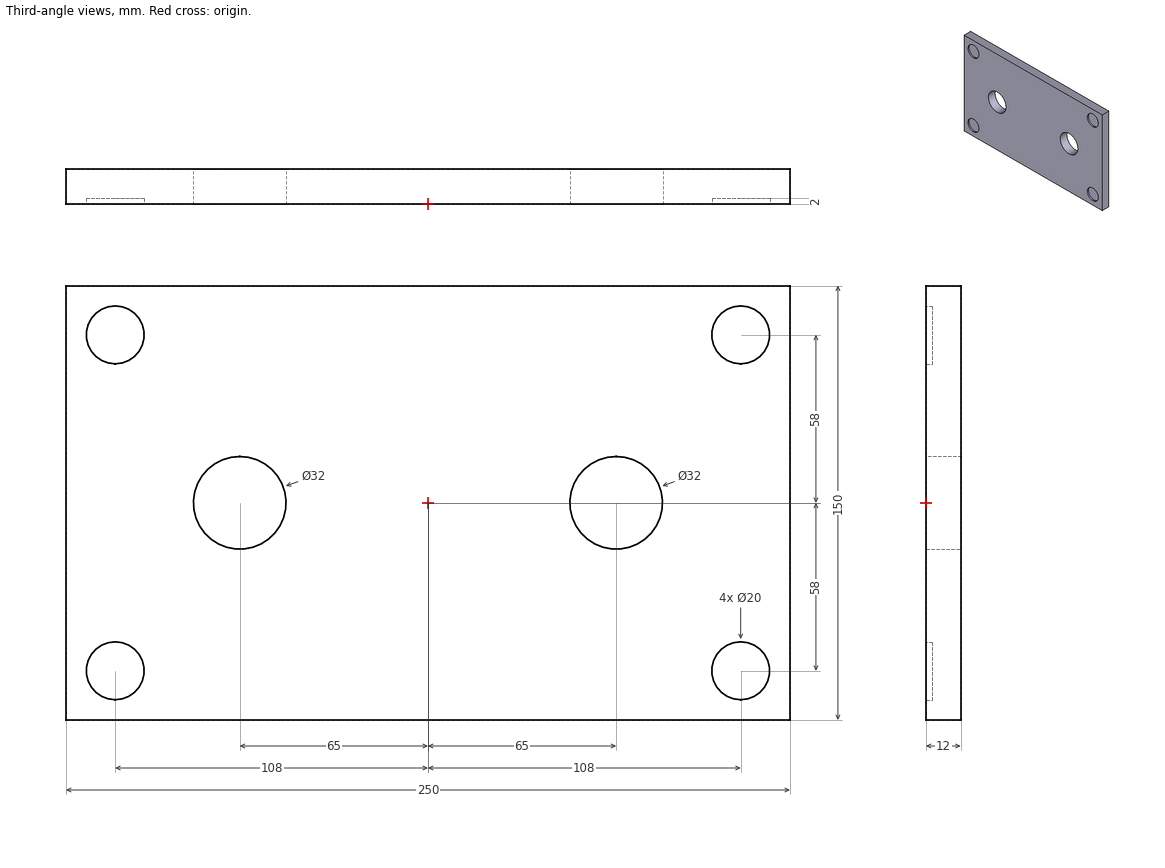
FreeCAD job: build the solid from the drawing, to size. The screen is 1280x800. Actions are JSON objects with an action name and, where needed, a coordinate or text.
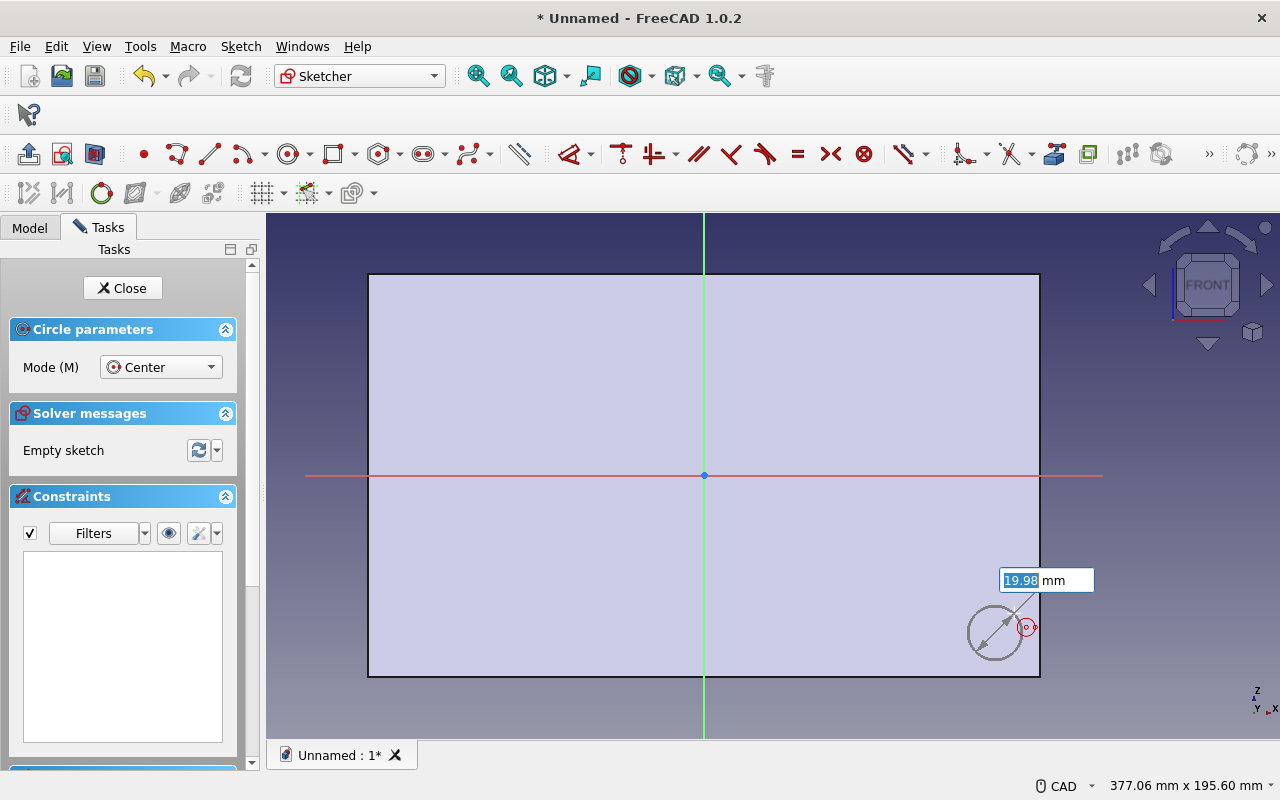
{"action": "type", "text": "20"}
{"action": "key", "text": "Return"}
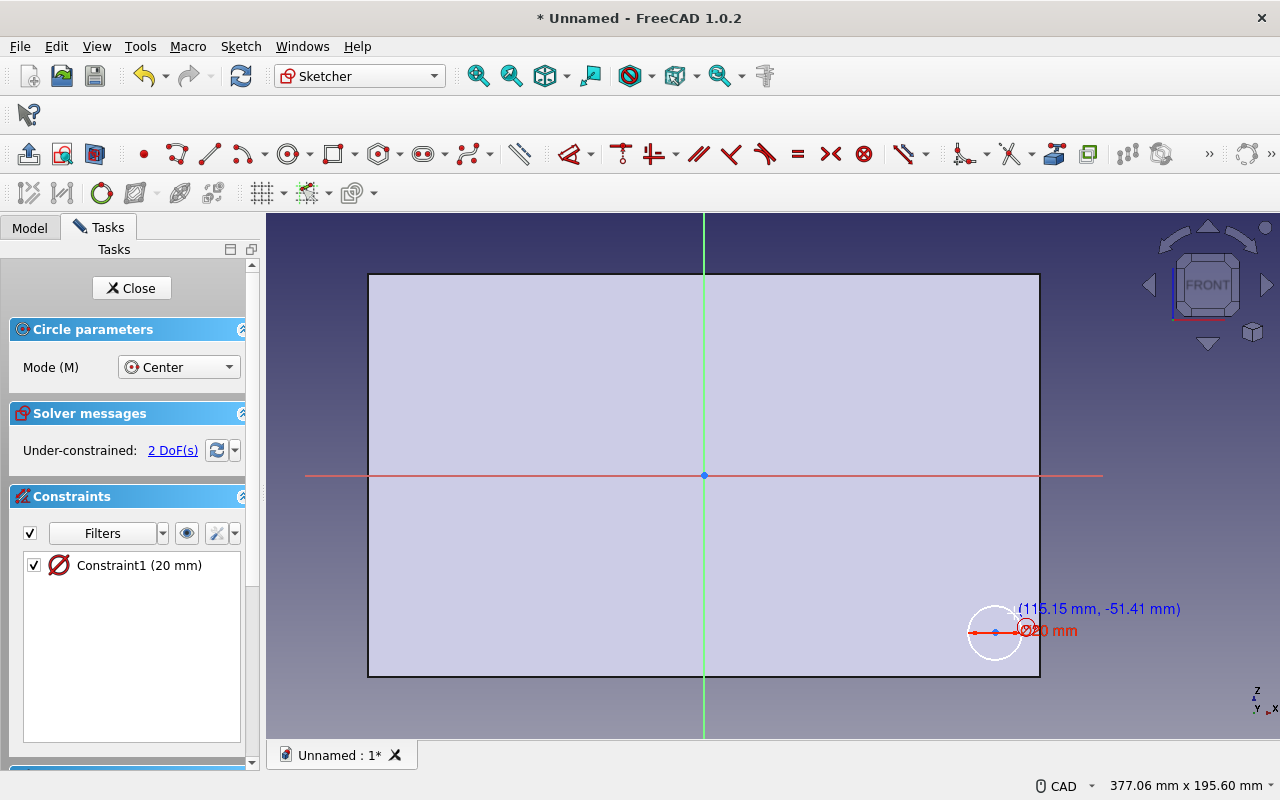
{"action": "left_click", "coordinate": [414, 632]}
{"action": "mouse_move", "coordinate": [433, 613]}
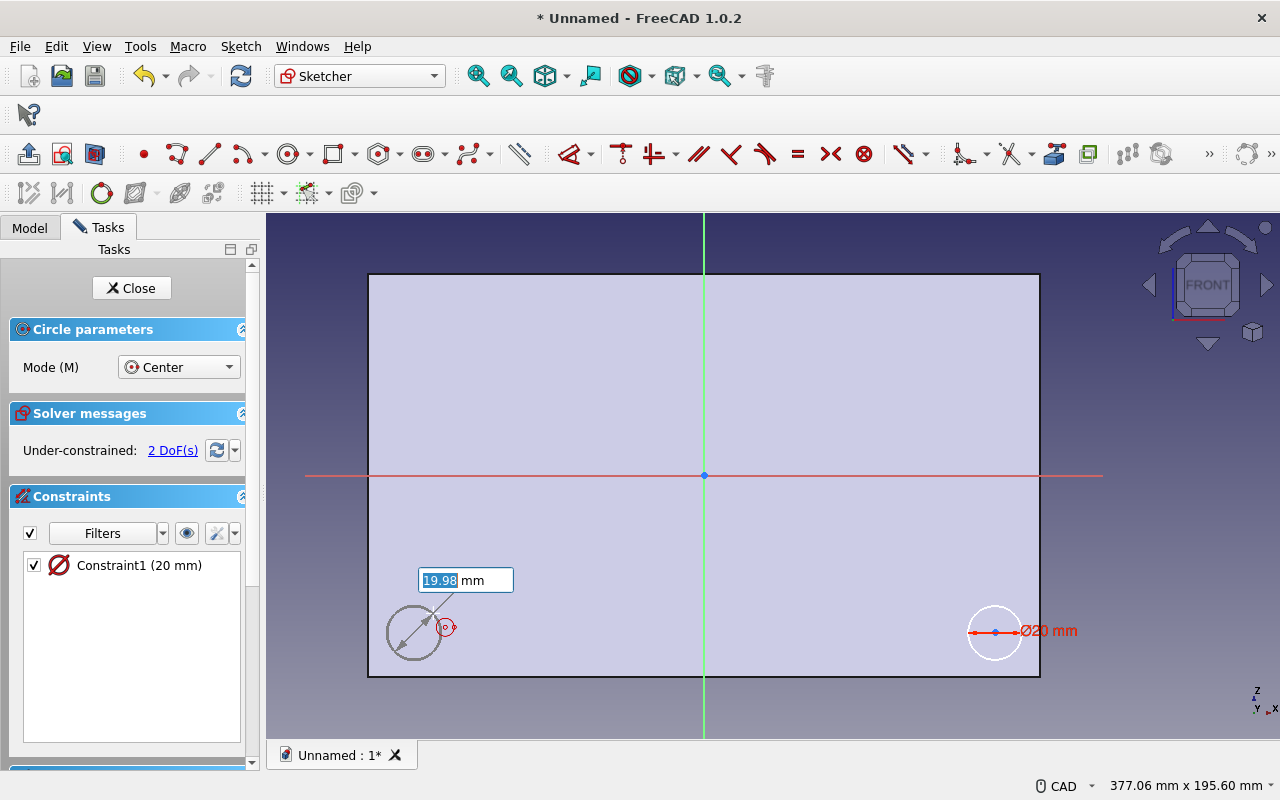
{"action": "type", "text": "20"}
{"action": "key", "text": "Return"}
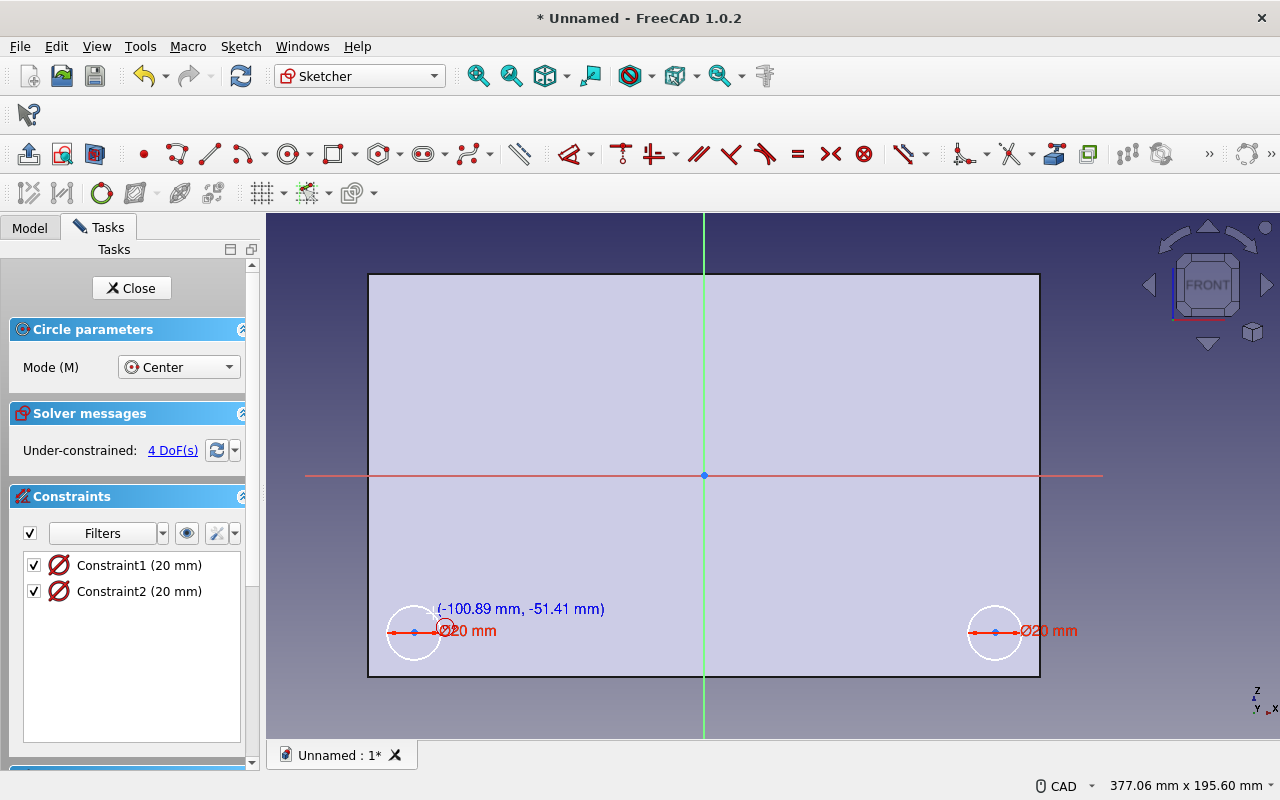
{"action": "left_click", "coordinate": [995, 320]}
{"action": "mouse_move", "coordinate": [1014, 301]}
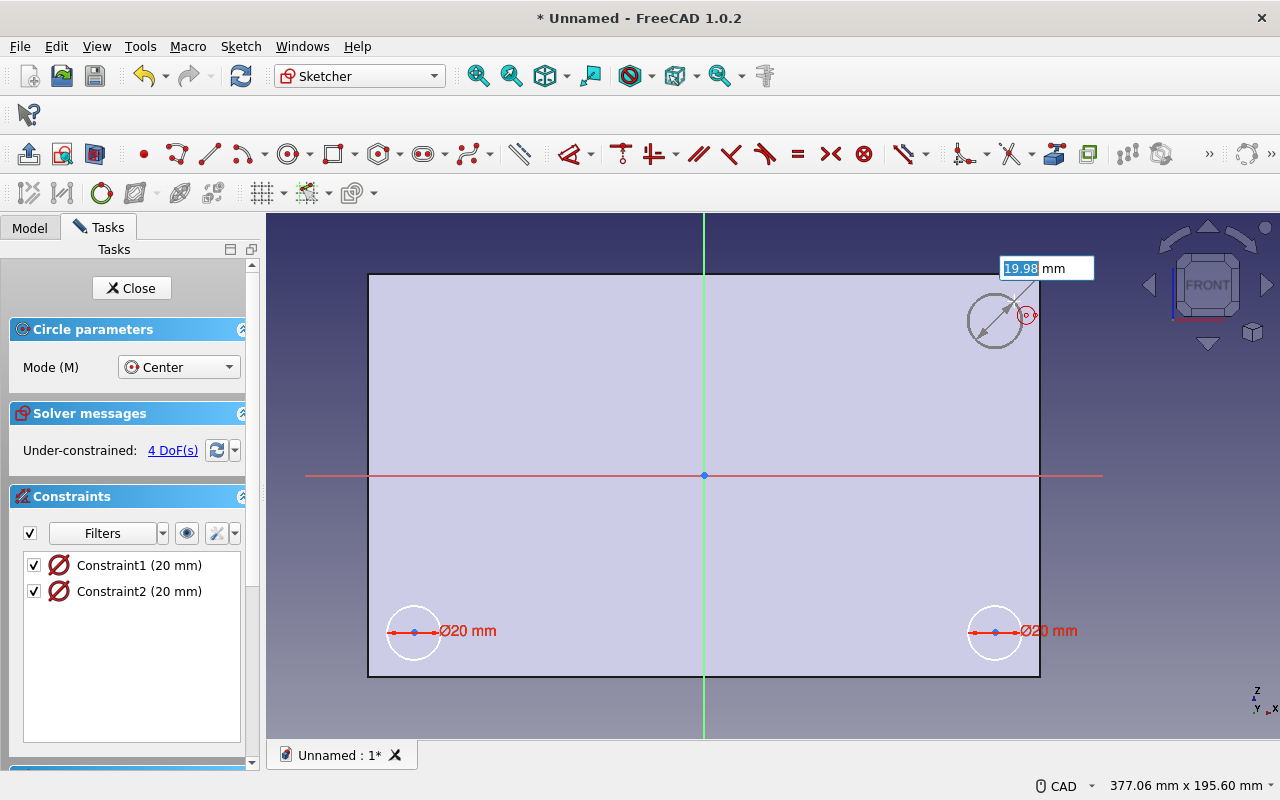
{"action": "type", "text": "20"}
{"action": "key", "text": "Return"}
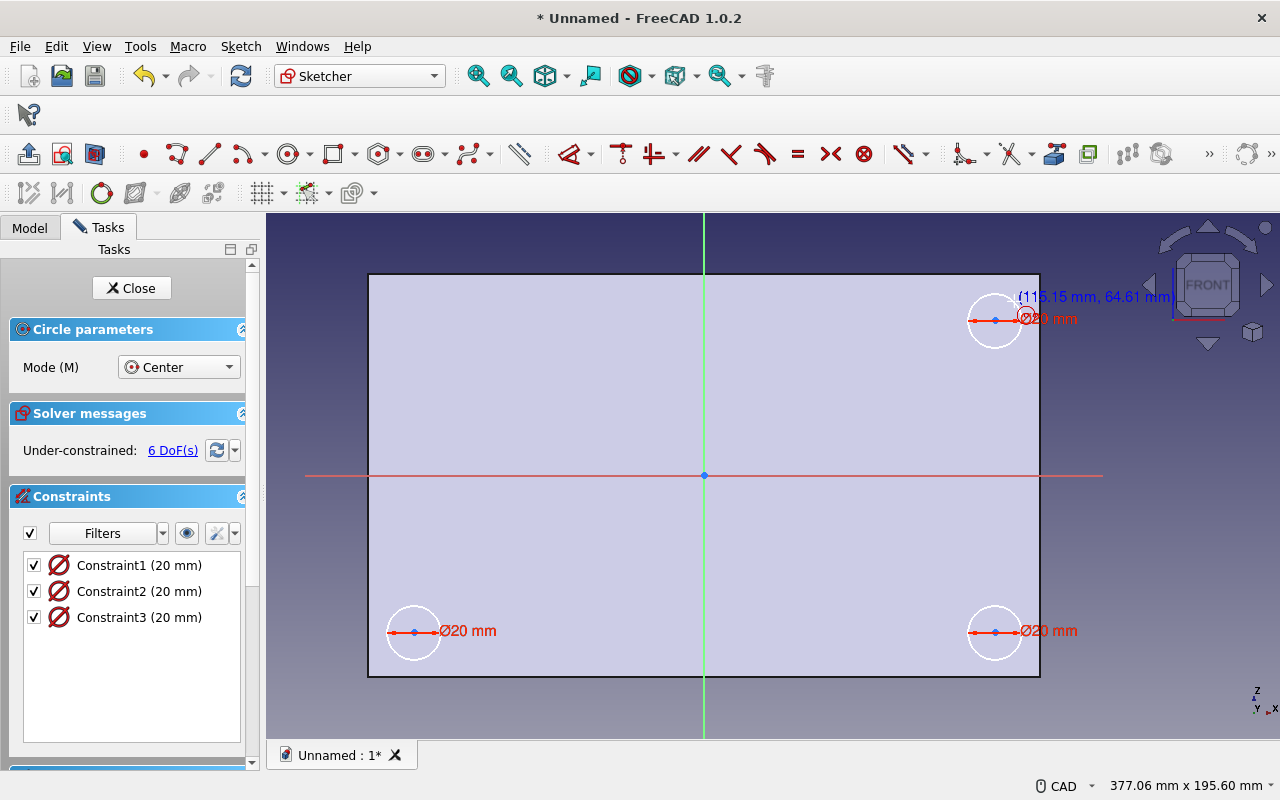
{"action": "left_click", "coordinate": [414, 320]}
{"action": "mouse_move", "coordinate": [433, 301]}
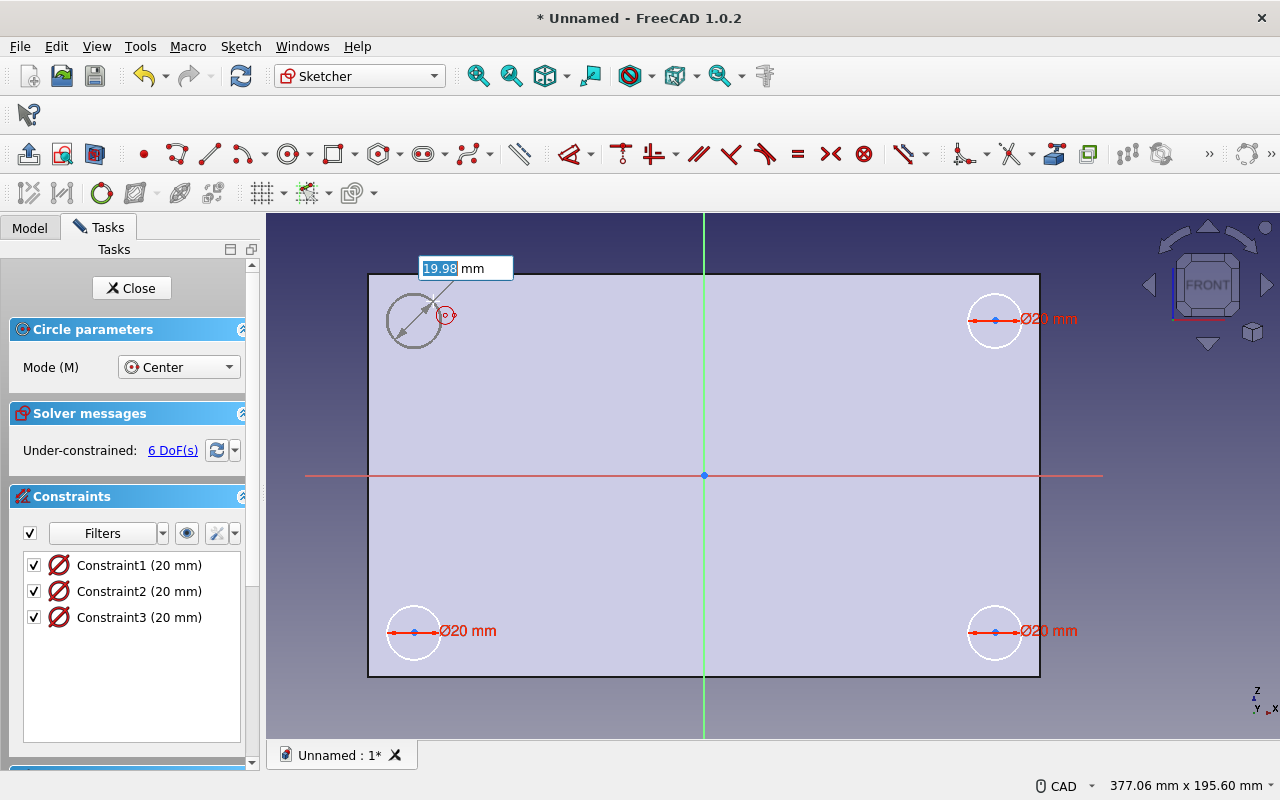
{"action": "type", "text": "20"}
{"action": "key", "text": "Return"}
{"action": "key", "text": "Escape"}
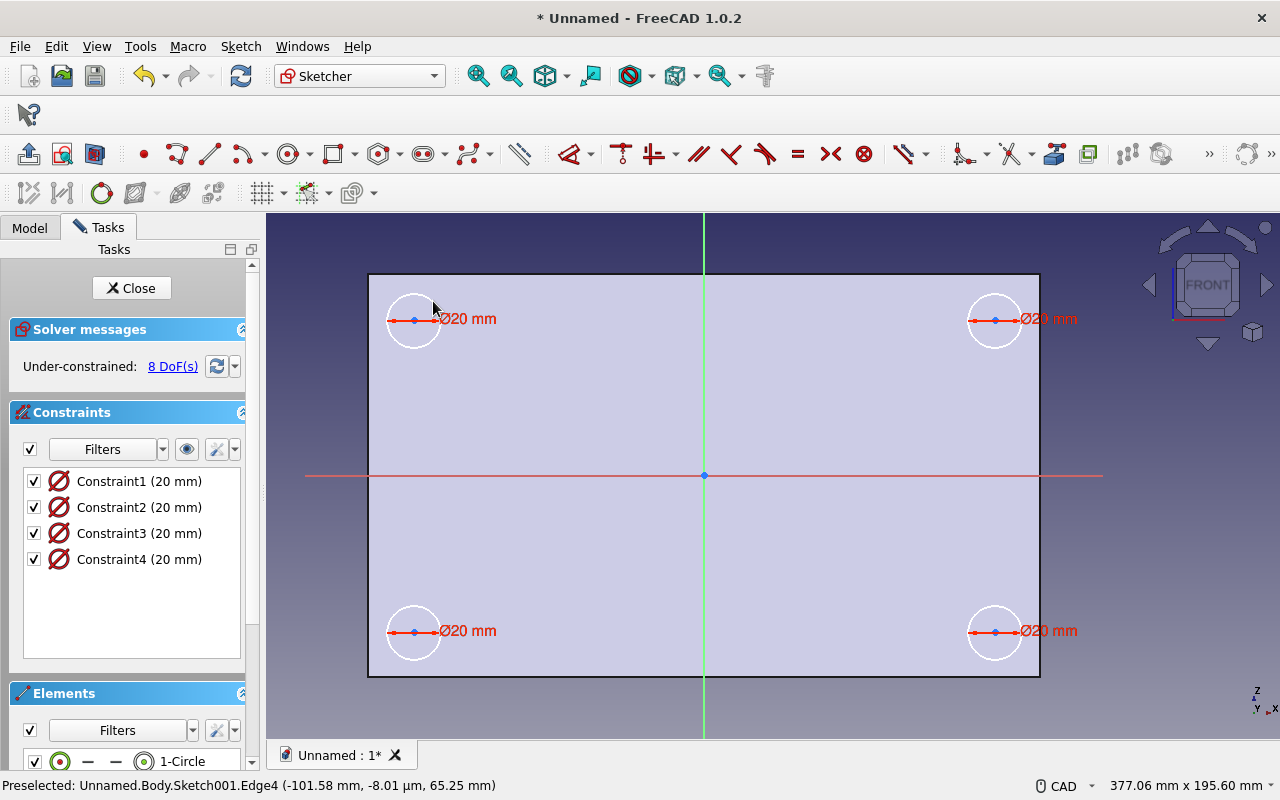
{"action": "left_click", "coordinate": [995, 633]}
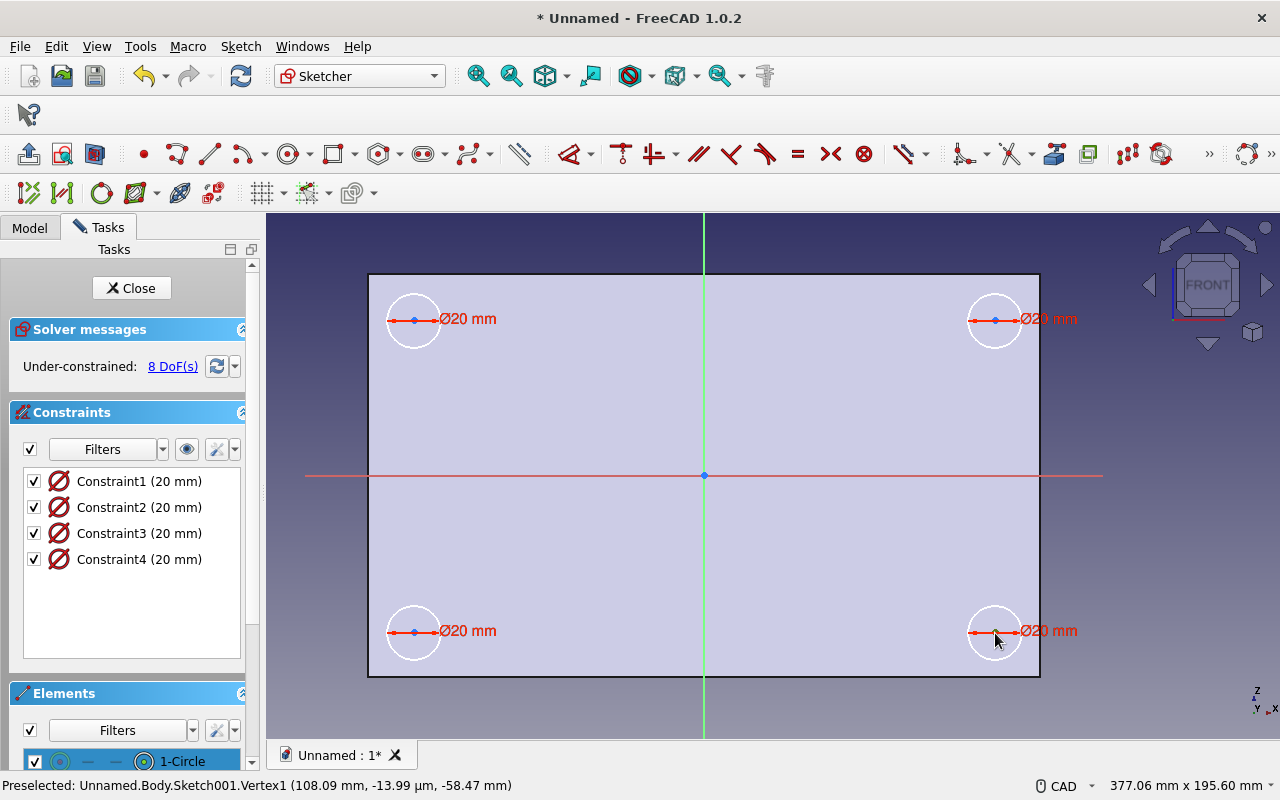
{"action": "left_click", "coordinate": [414, 633]}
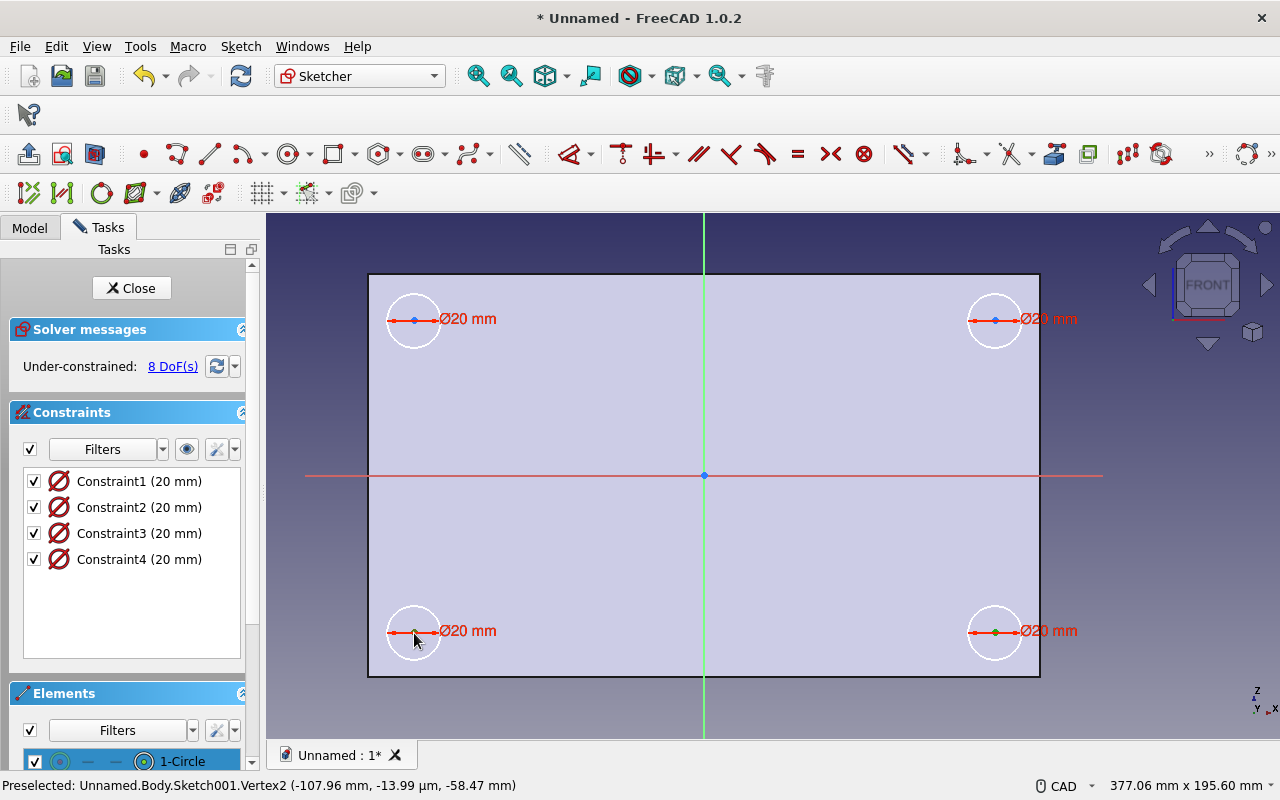
{"action": "key", "text": "h"}